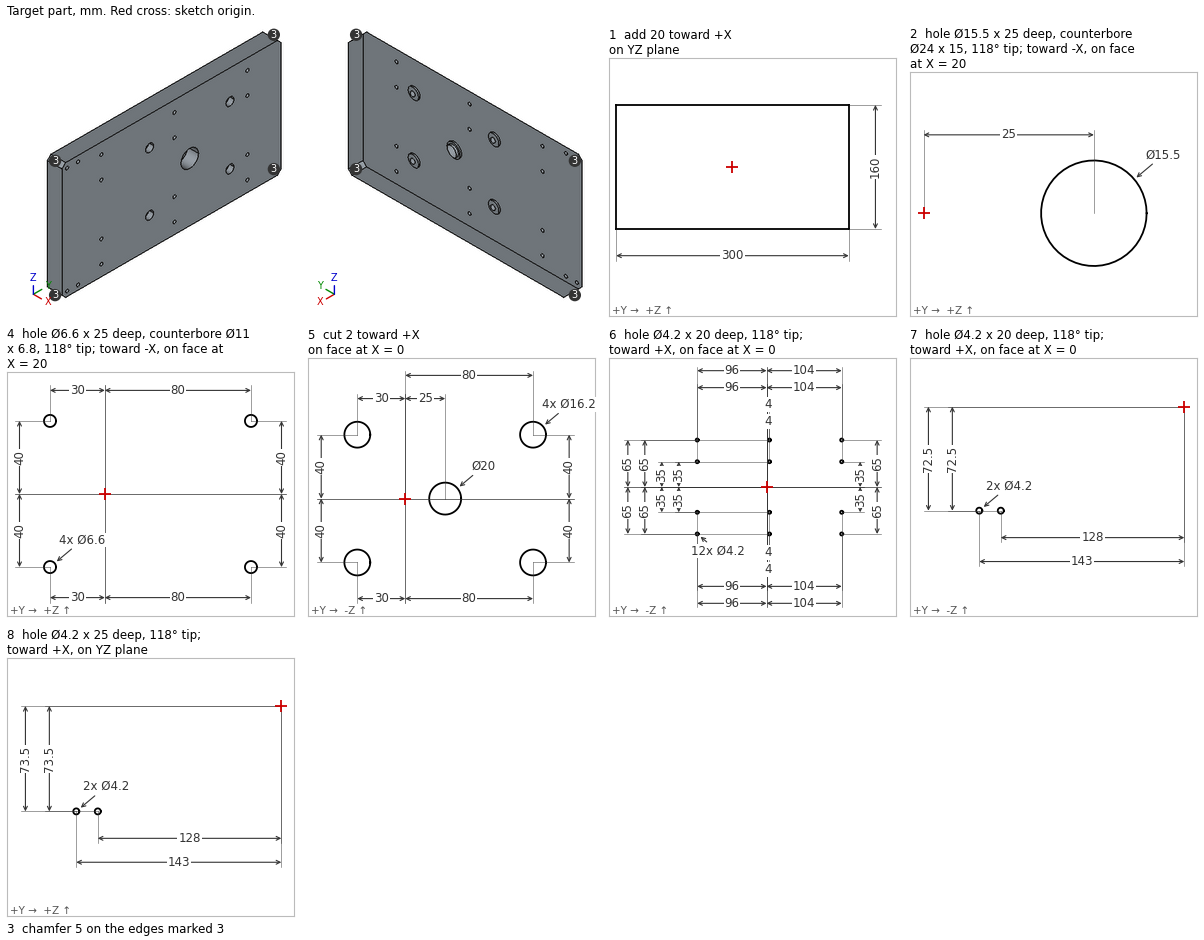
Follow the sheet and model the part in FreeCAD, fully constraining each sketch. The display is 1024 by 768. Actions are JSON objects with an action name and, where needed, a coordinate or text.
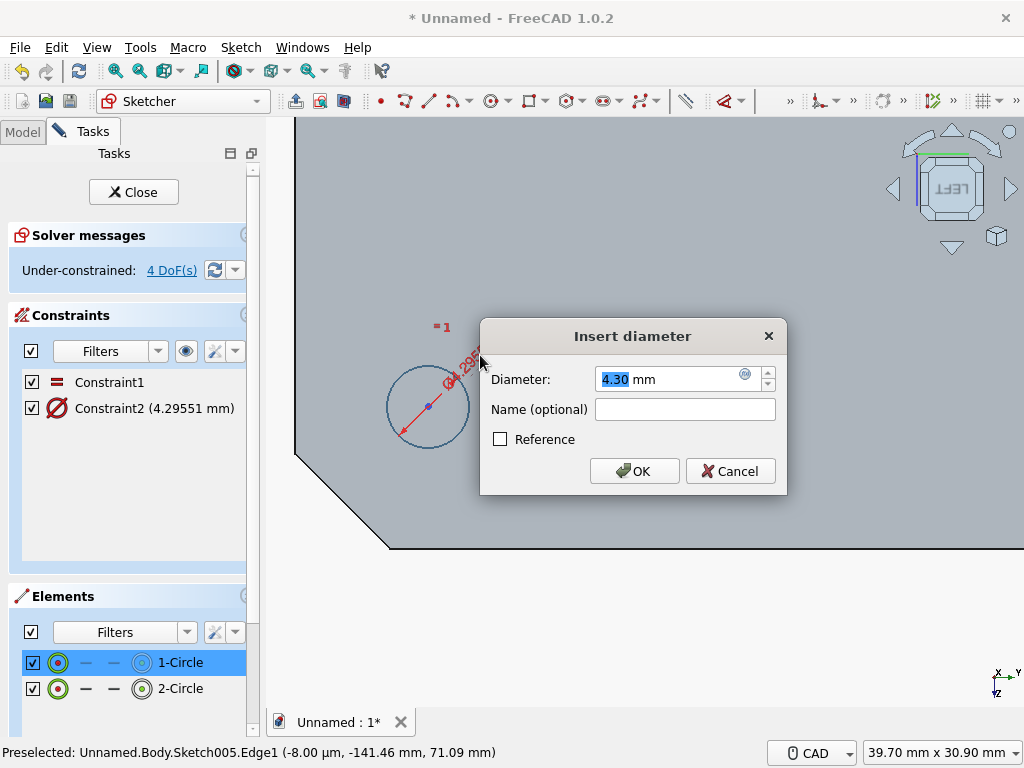
{"action": "type", "text": "4.2"}
{"action": "key", "text": "Return"}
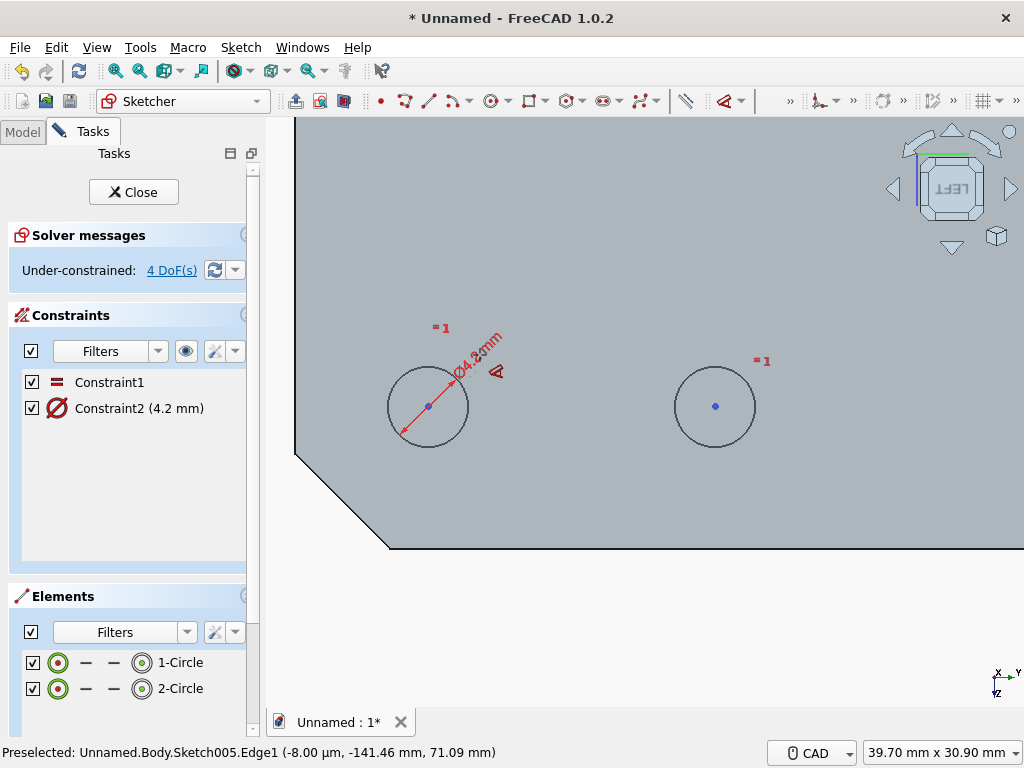
{"action": "left_click", "coordinate": [428, 407]}
{"action": "left_click", "coordinate": [644, 441]}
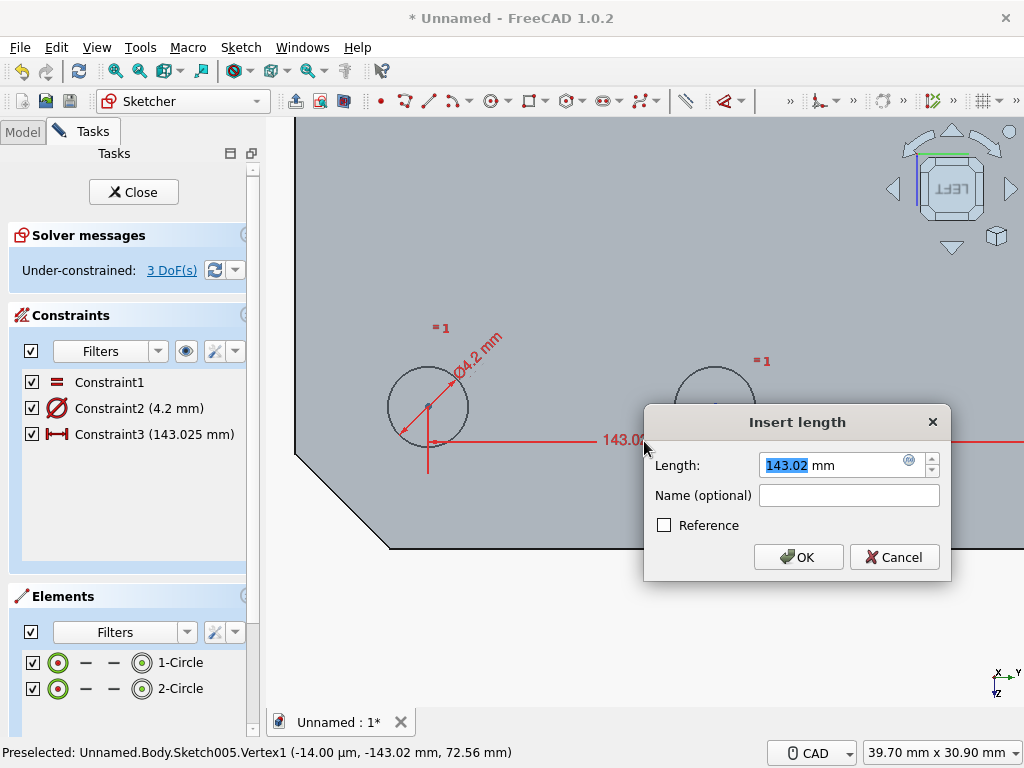
{"action": "type", "text": "143"}
{"action": "key", "text": "Return"}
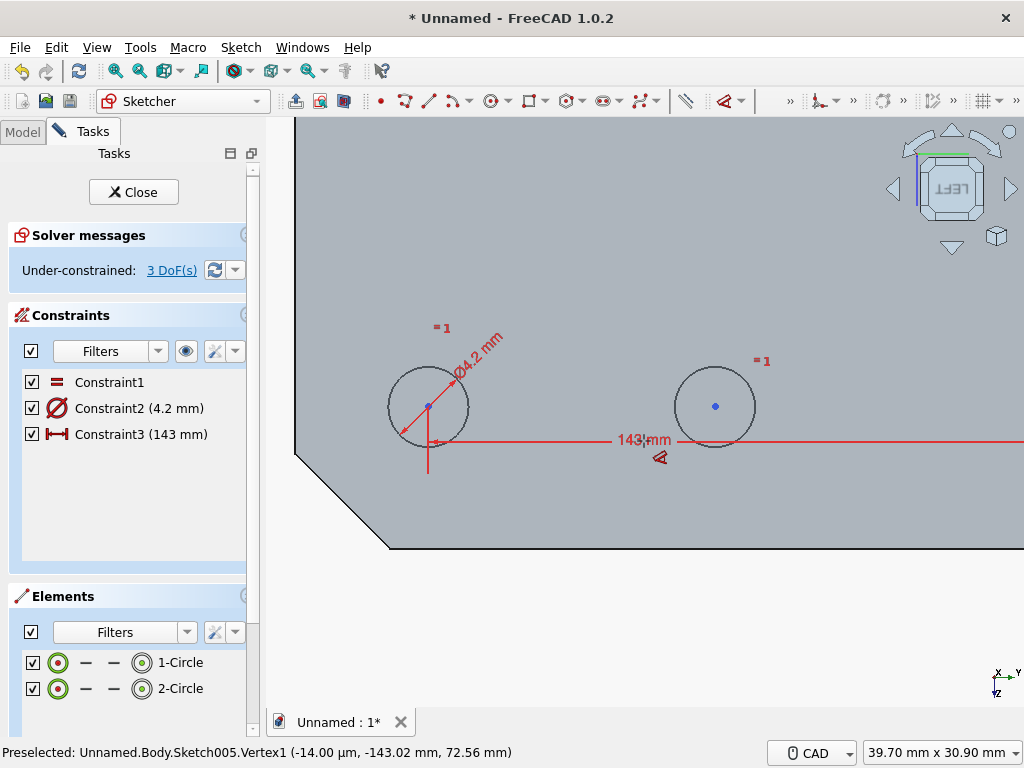
{"action": "left_click", "coordinate": [715, 407]}
{"action": "left_click", "coordinate": [787, 441]}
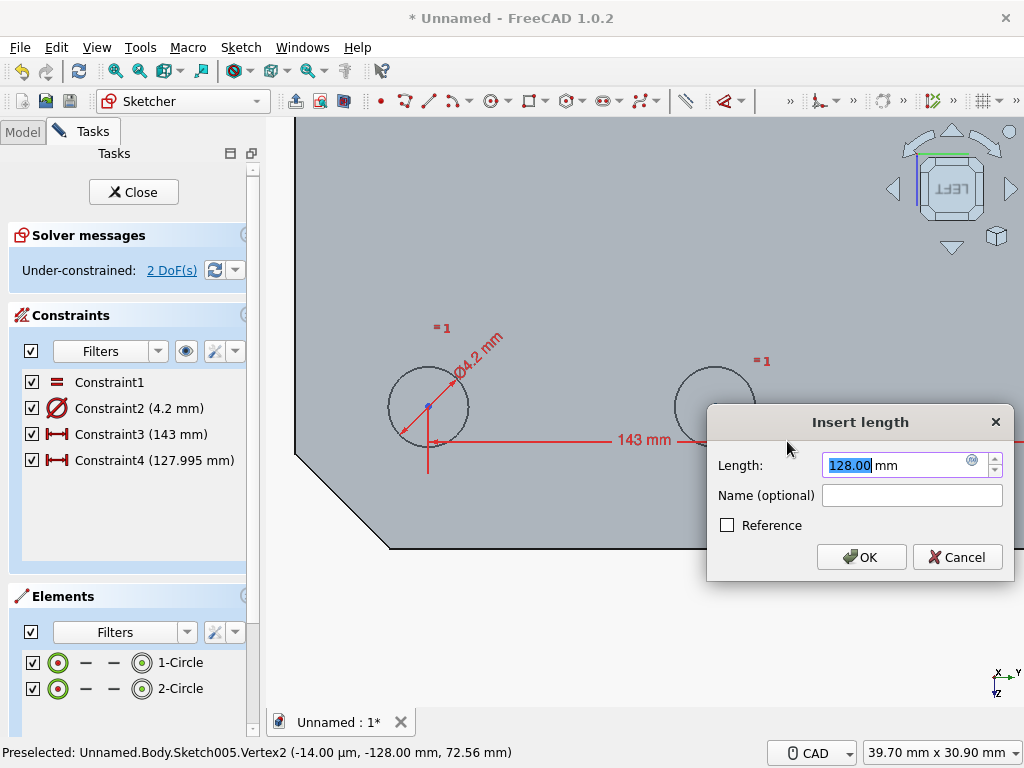
{"action": "type", "text": "128"}
{"action": "key", "text": "Return"}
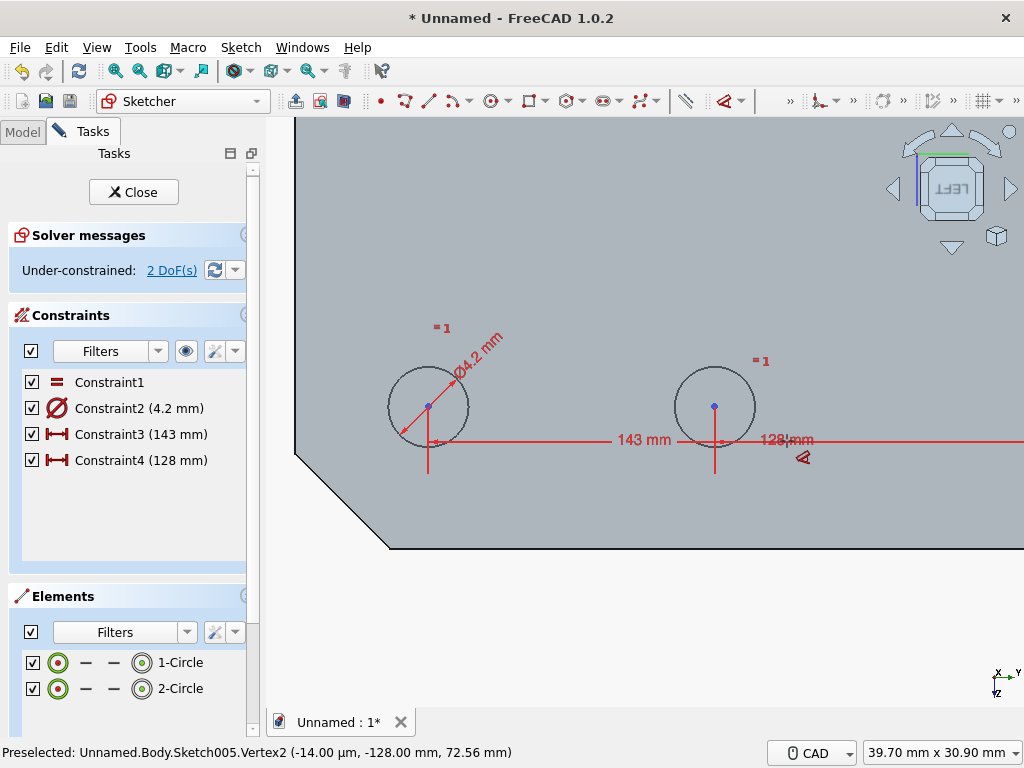
{"action": "left_click", "coordinate": [428, 407]}
{"action": "left_click", "coordinate": [394, 276]}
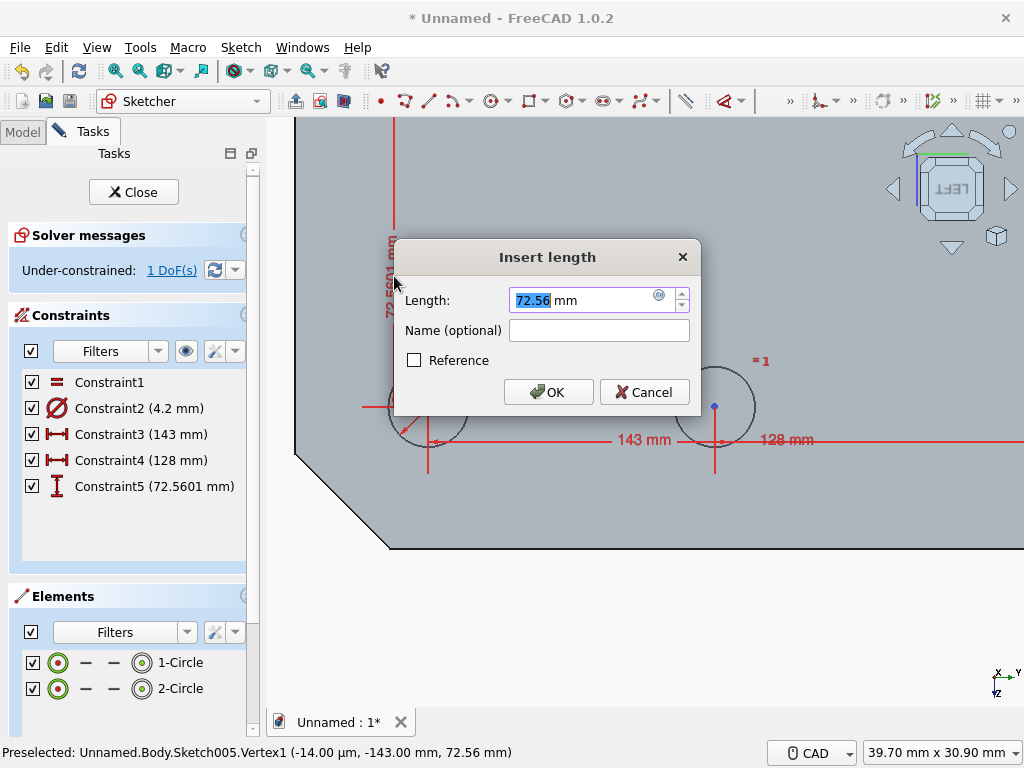
{"action": "type", "text": "72.5"}
{"action": "key", "text": "Return"}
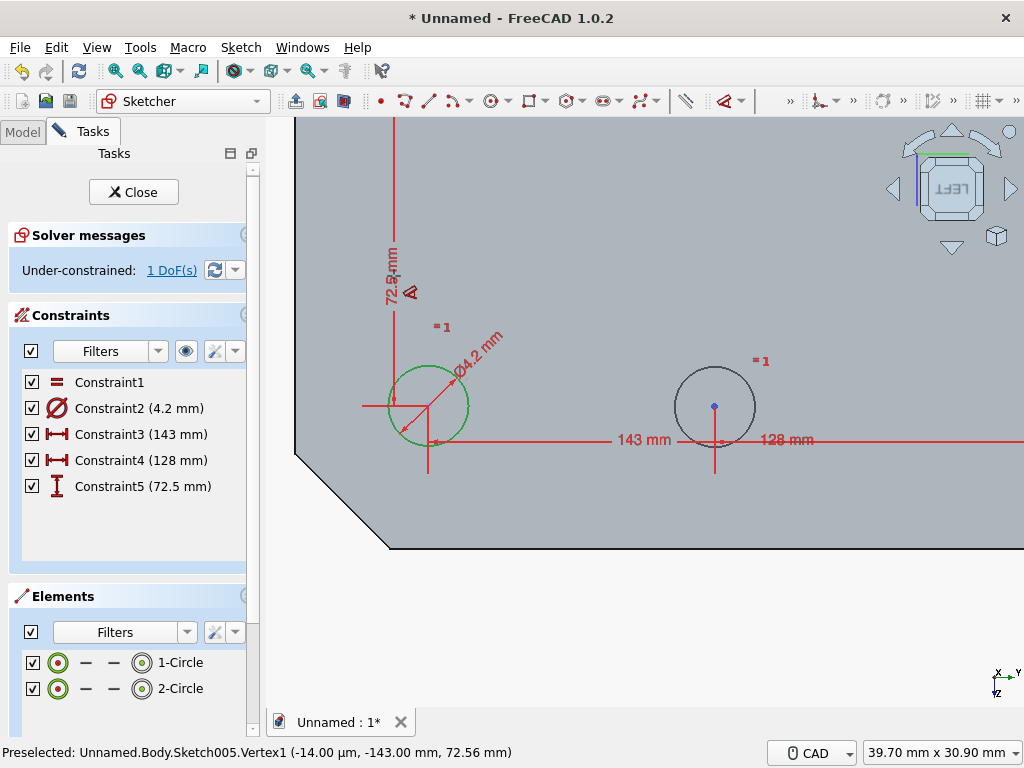
{"action": "left_click", "coordinate": [715, 407]}
{"action": "left_click", "coordinate": [681, 276]}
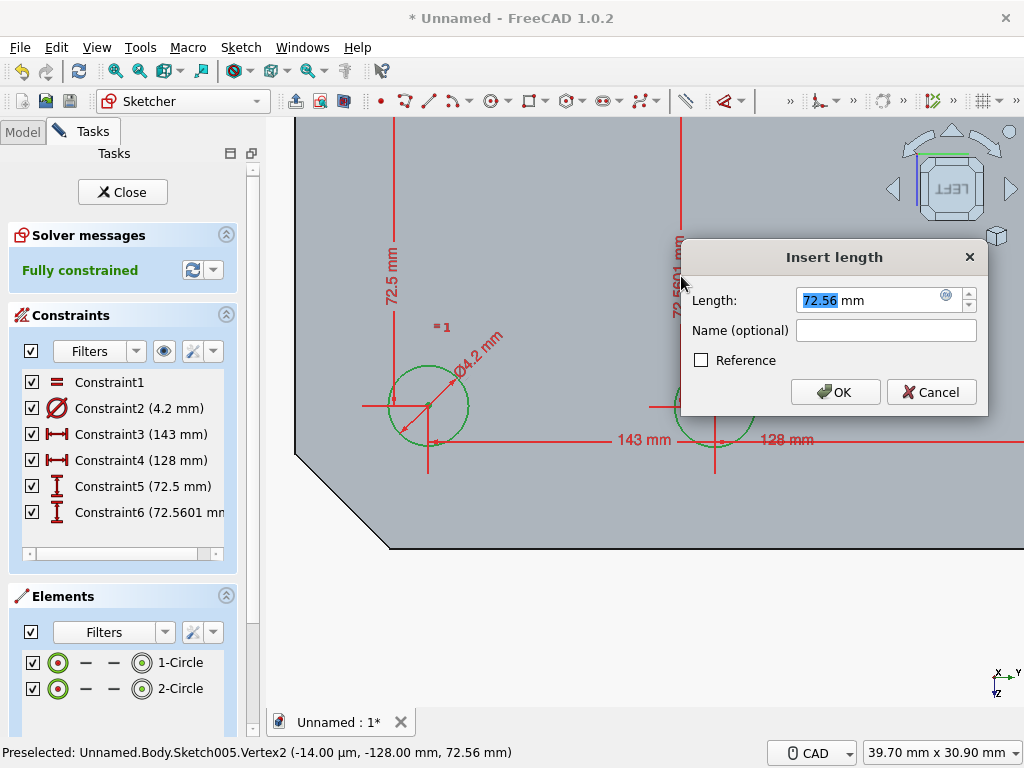
{"action": "type", "text": "72.5"}
{"action": "key", "text": "Return"}
{"action": "key", "text": "Escape"}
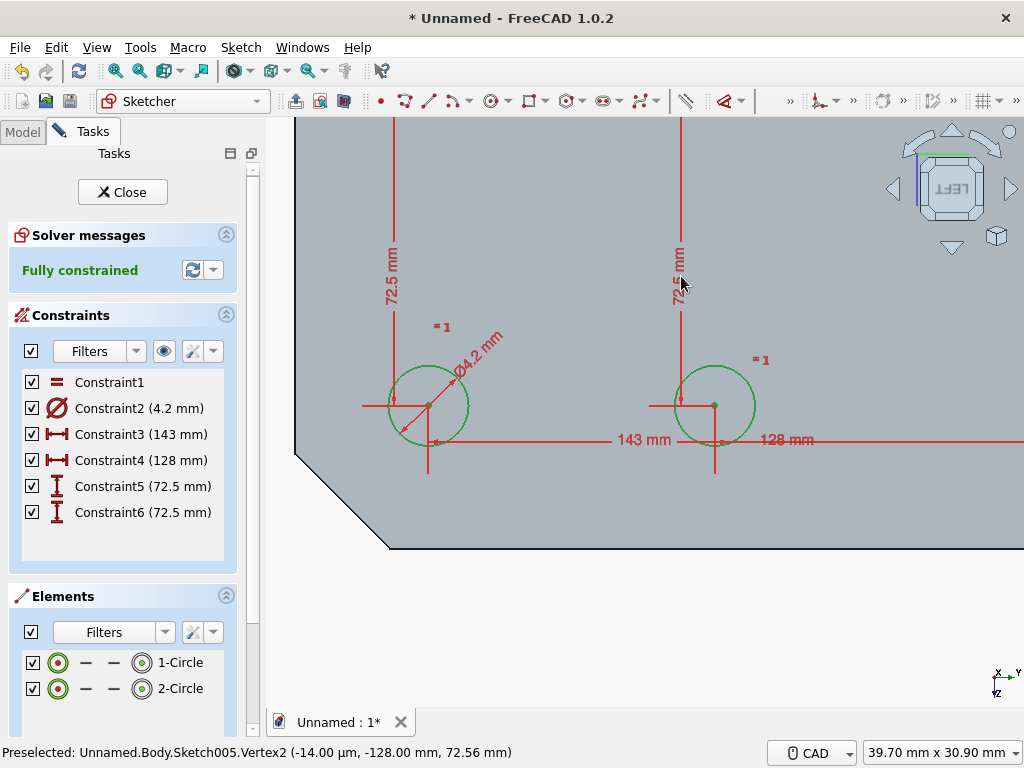
{"action": "left_click", "coordinate": [123, 192]}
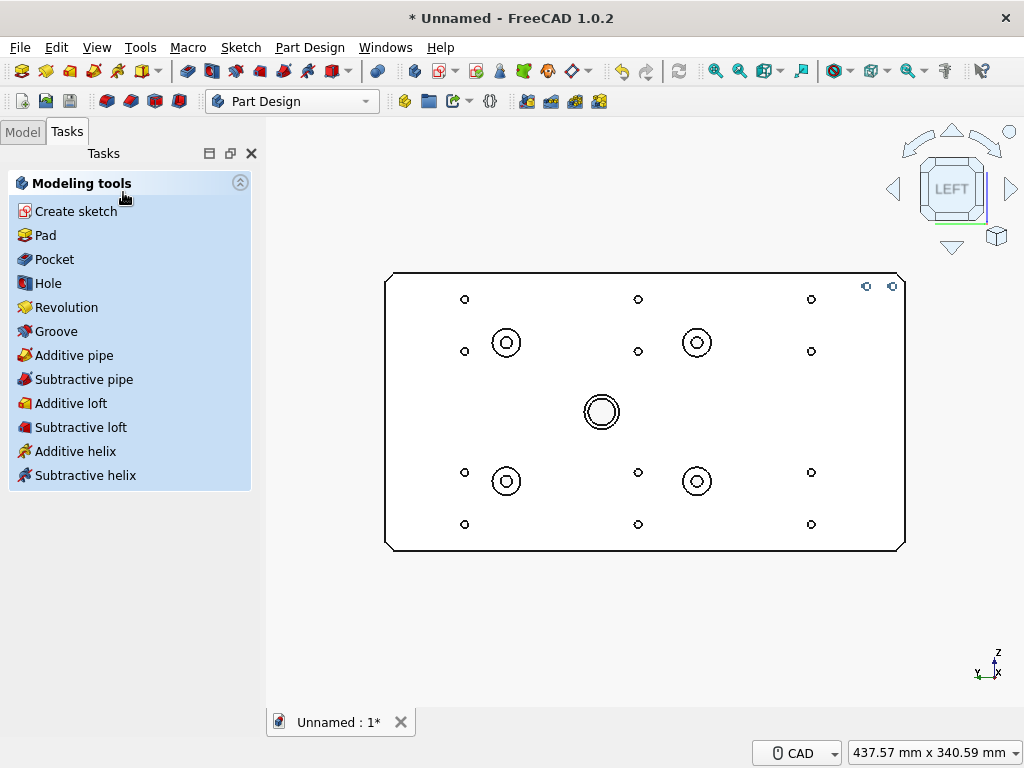
{"action": "left_click", "coordinate": [212, 72]}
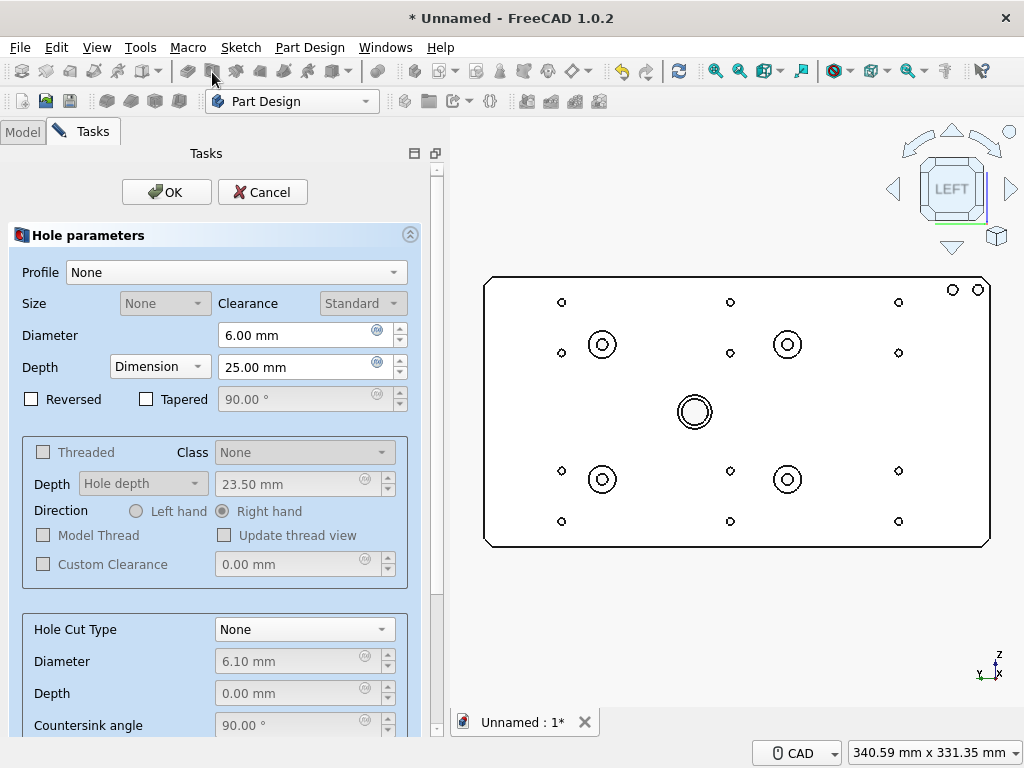
{"action": "triple_click", "coordinate": [305, 335]}